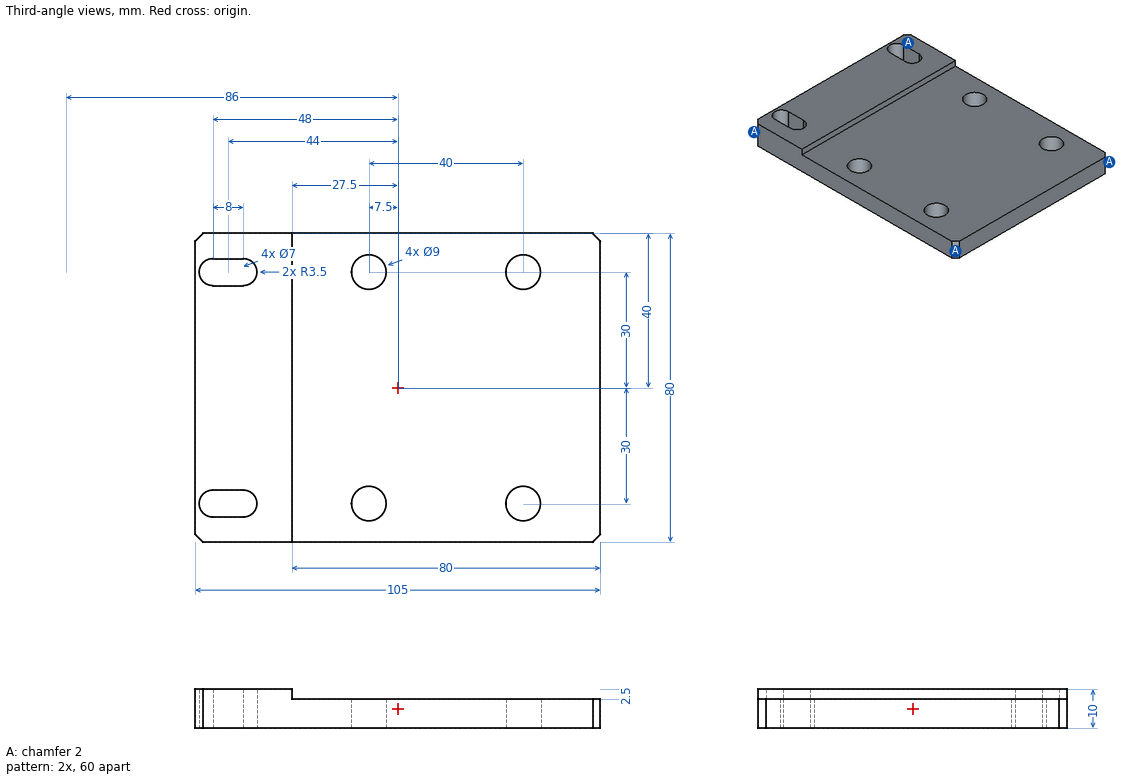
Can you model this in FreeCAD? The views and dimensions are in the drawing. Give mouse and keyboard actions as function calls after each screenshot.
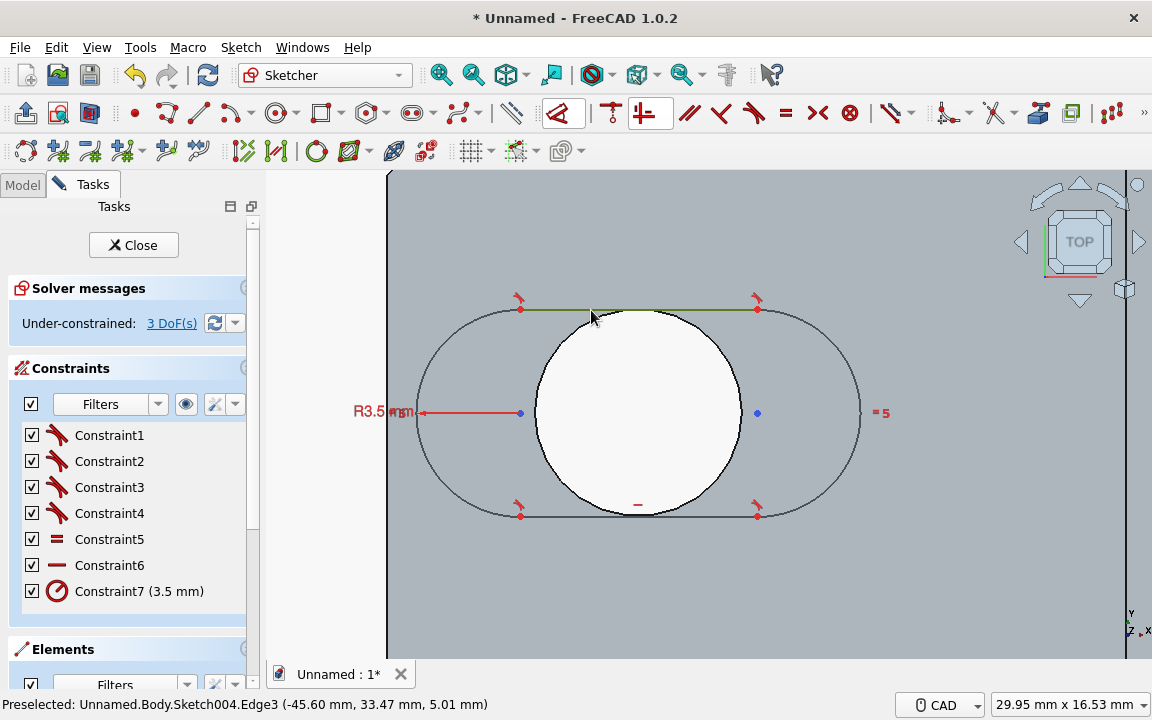
key(l)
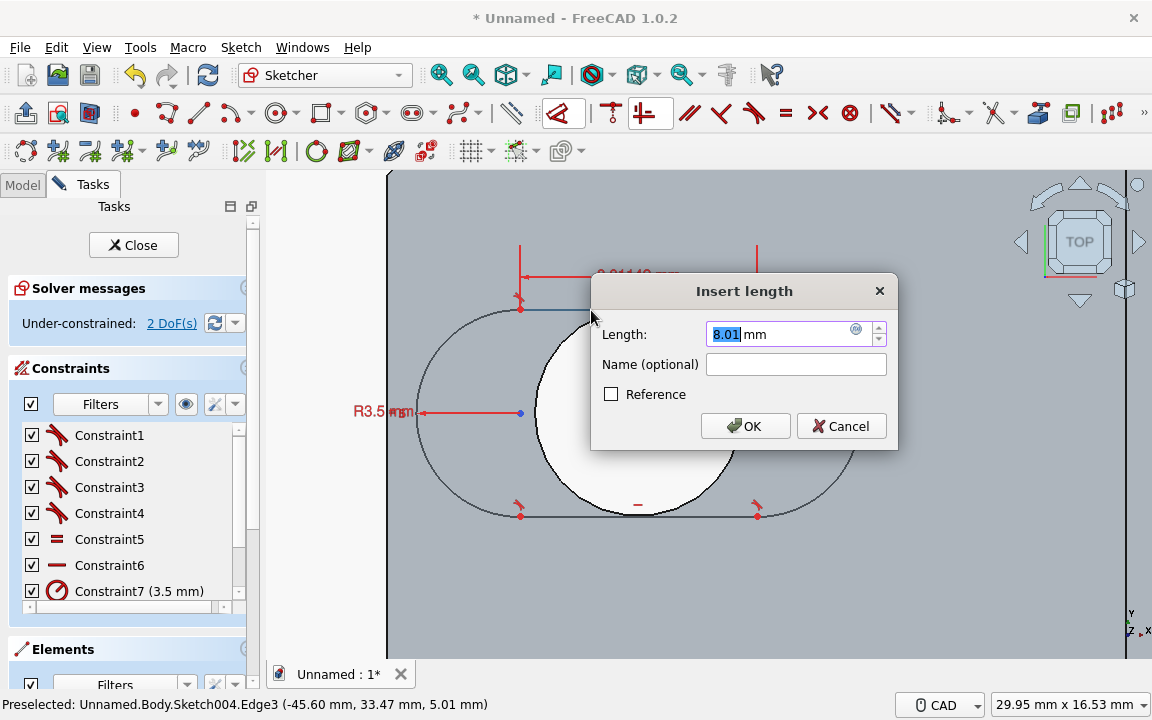
text(8)
key(Return)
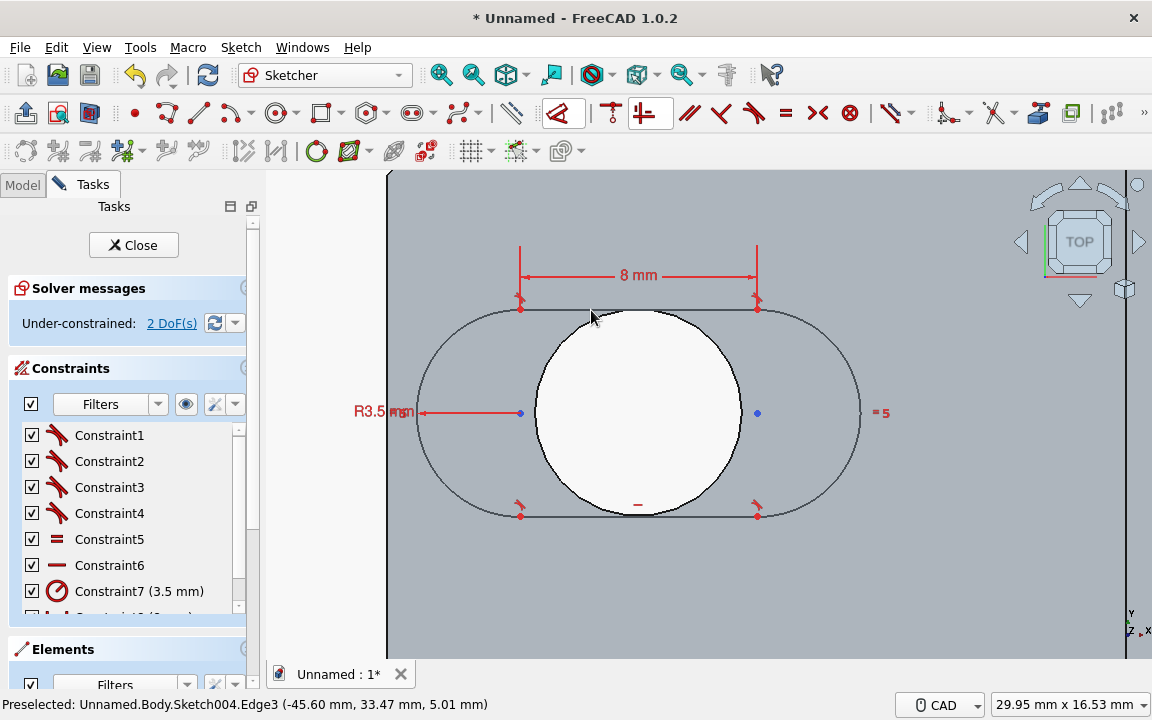
click(520, 310)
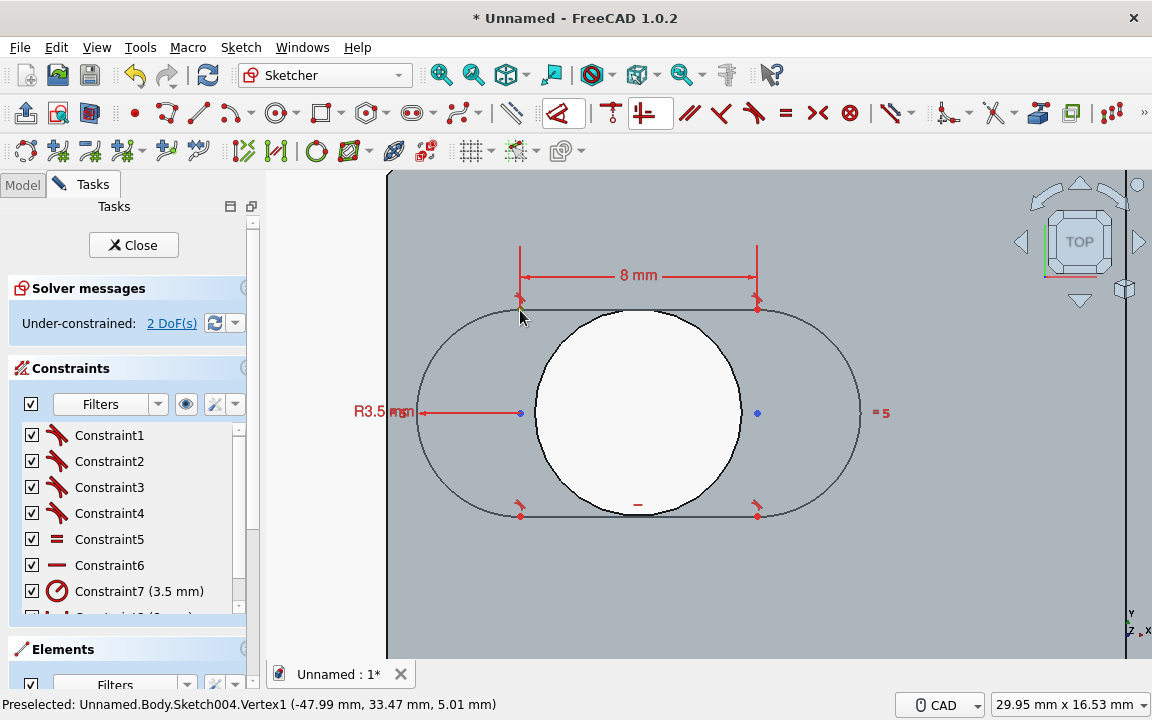
key(l)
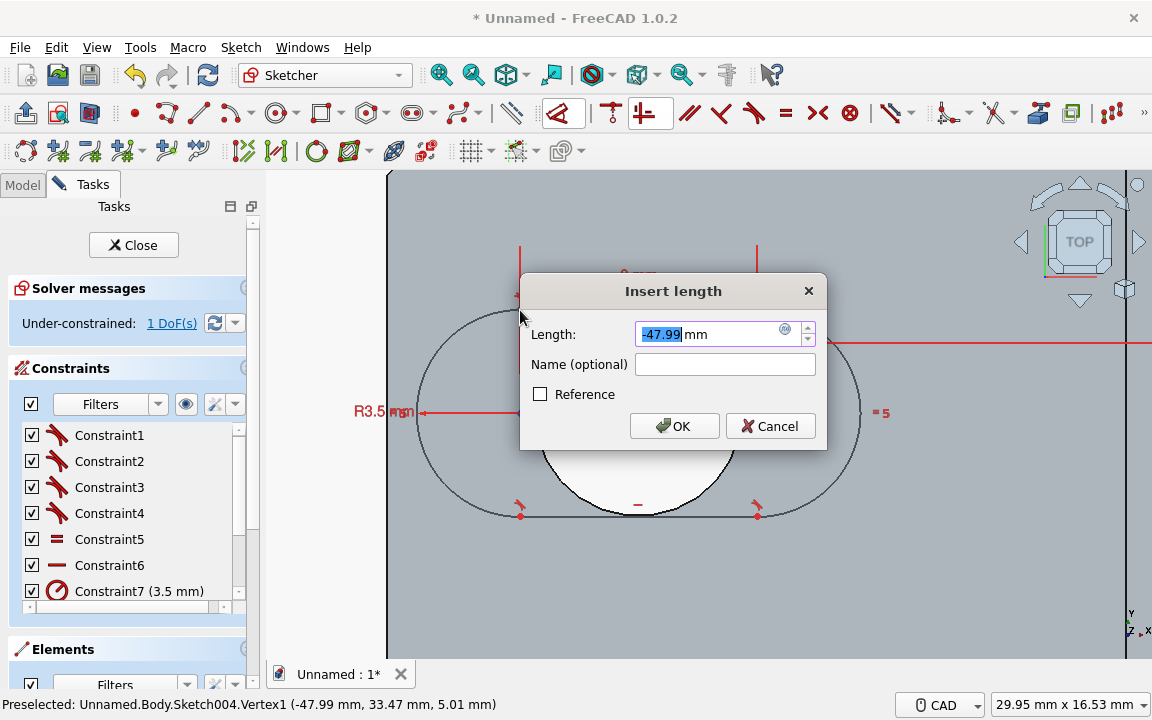
text(-48)
key(Return)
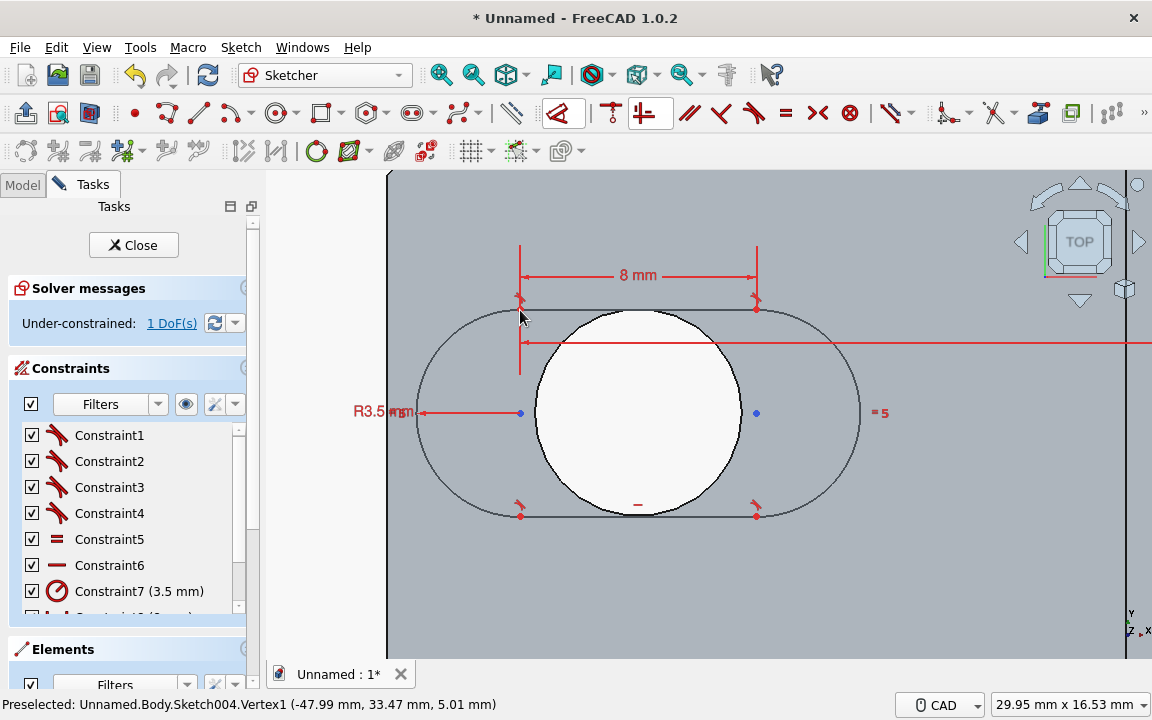
click(520, 413)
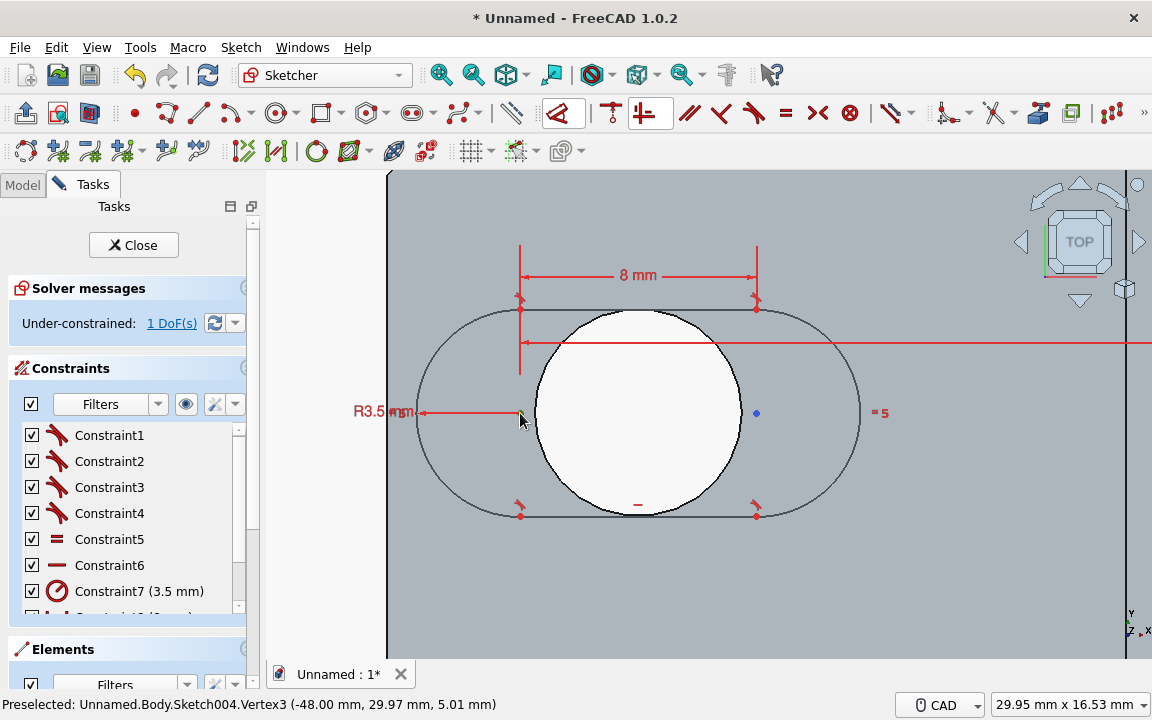
key(i)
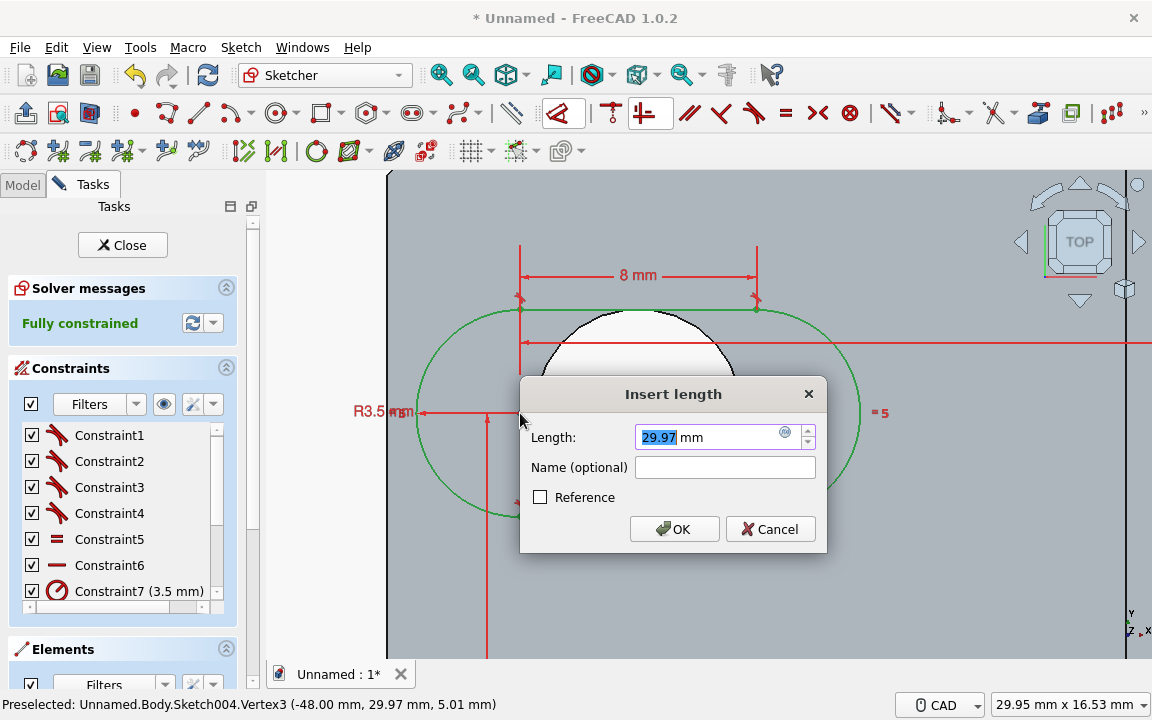
text(30)
key(Return)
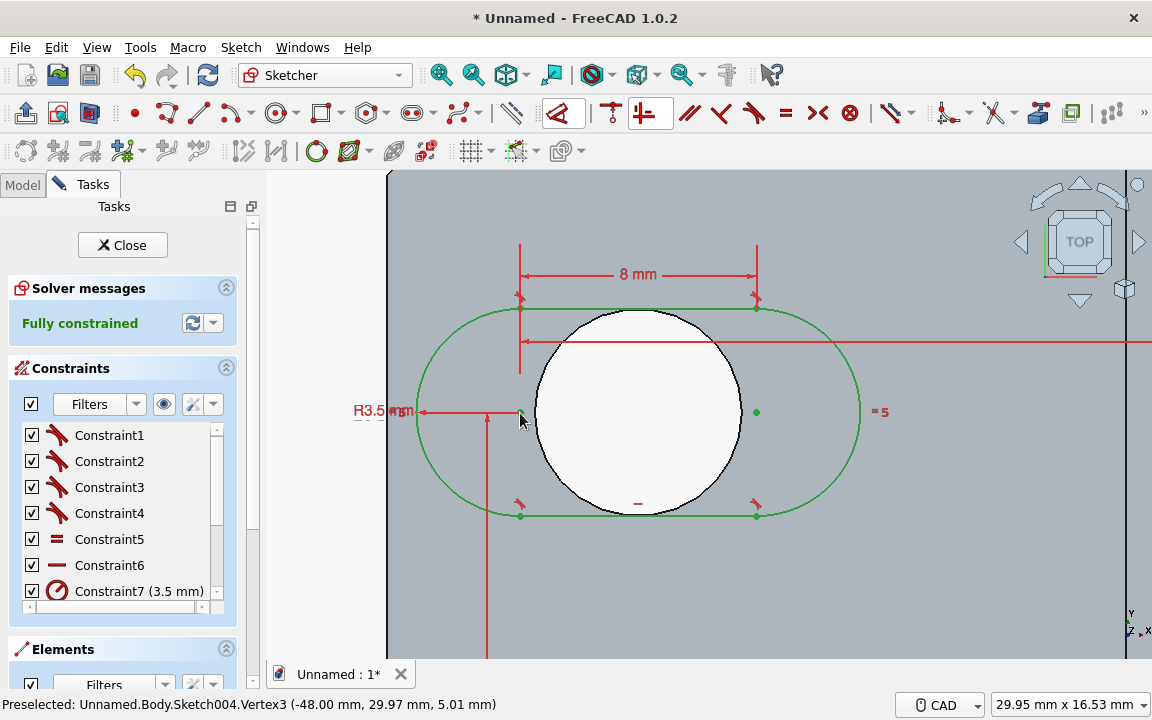
click(123, 245)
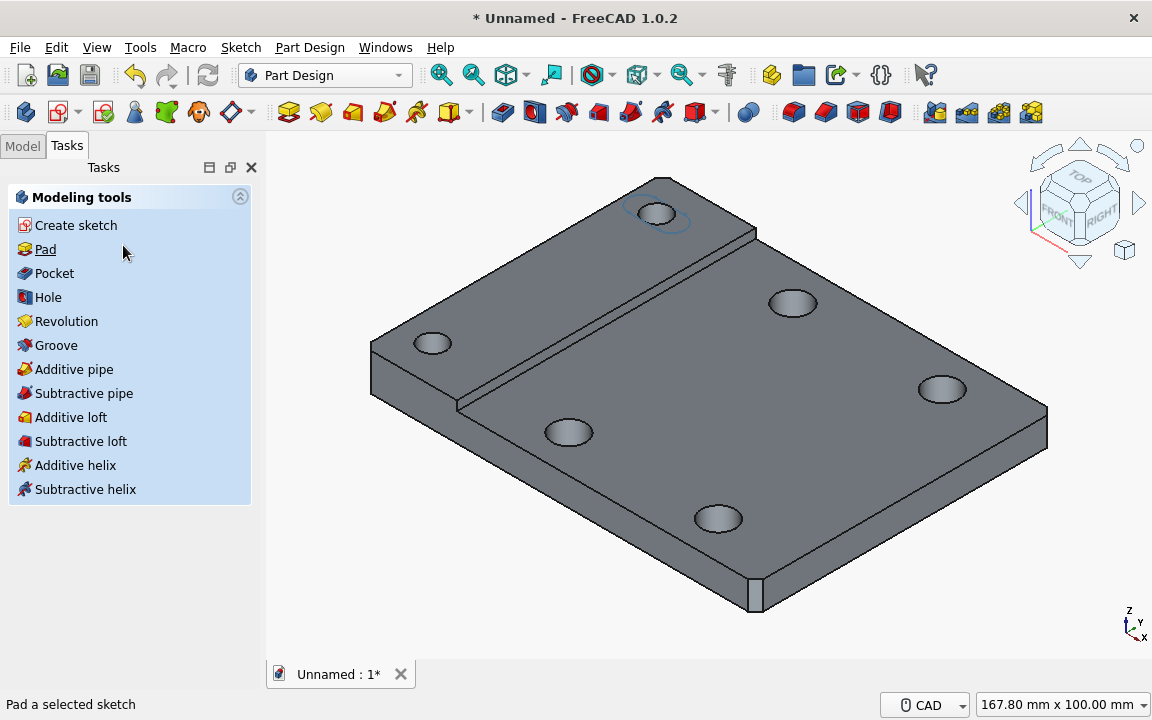
click(504, 112)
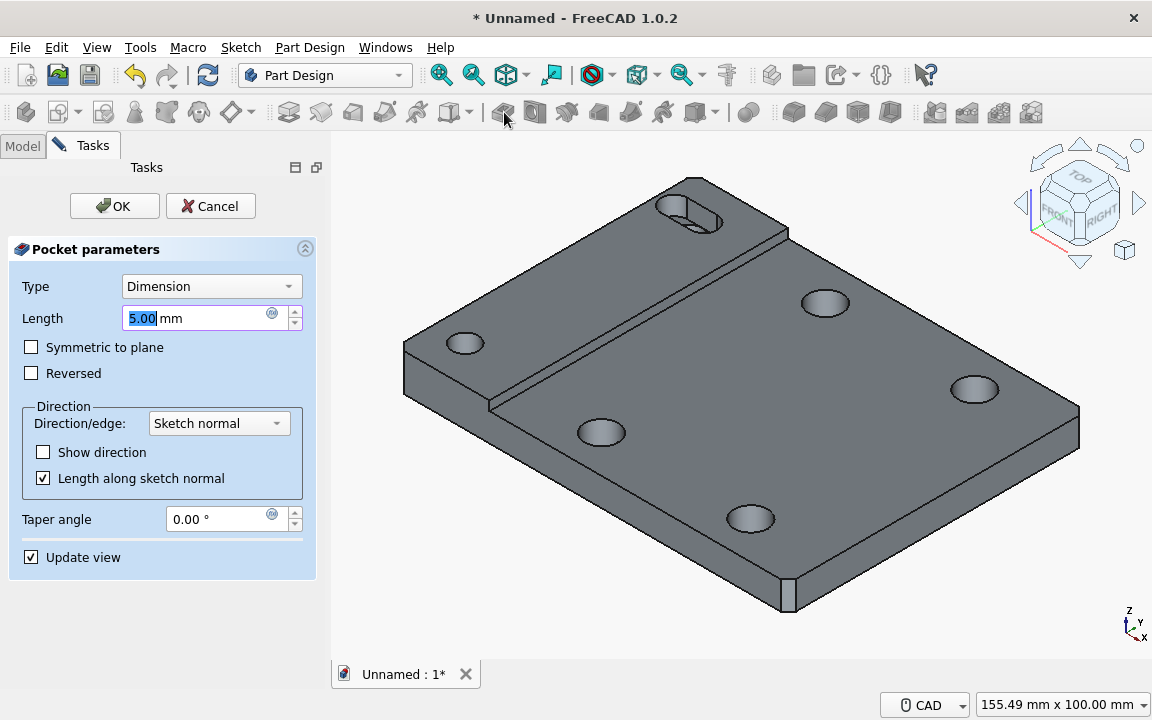
text(10)
key(Tab)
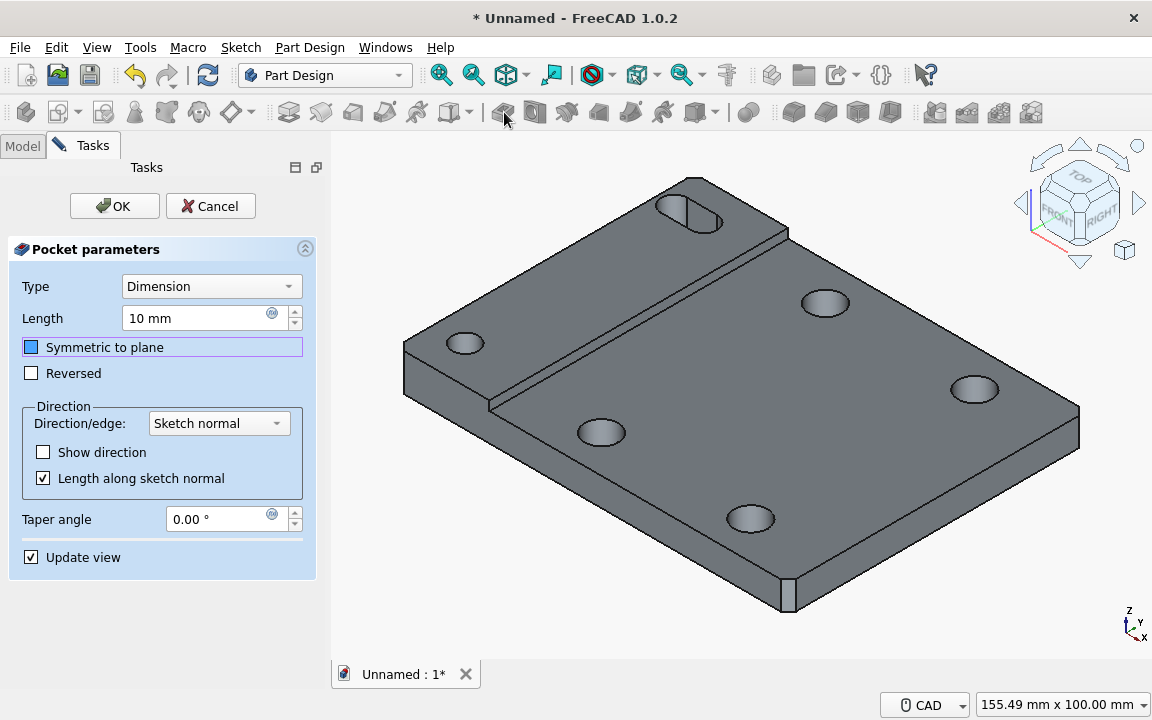
click(115, 206)